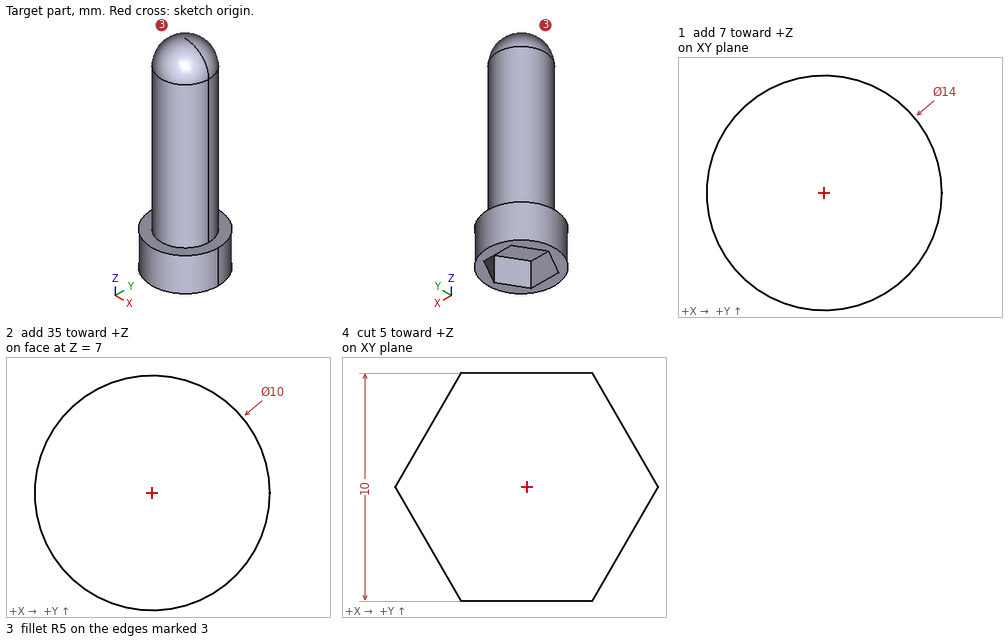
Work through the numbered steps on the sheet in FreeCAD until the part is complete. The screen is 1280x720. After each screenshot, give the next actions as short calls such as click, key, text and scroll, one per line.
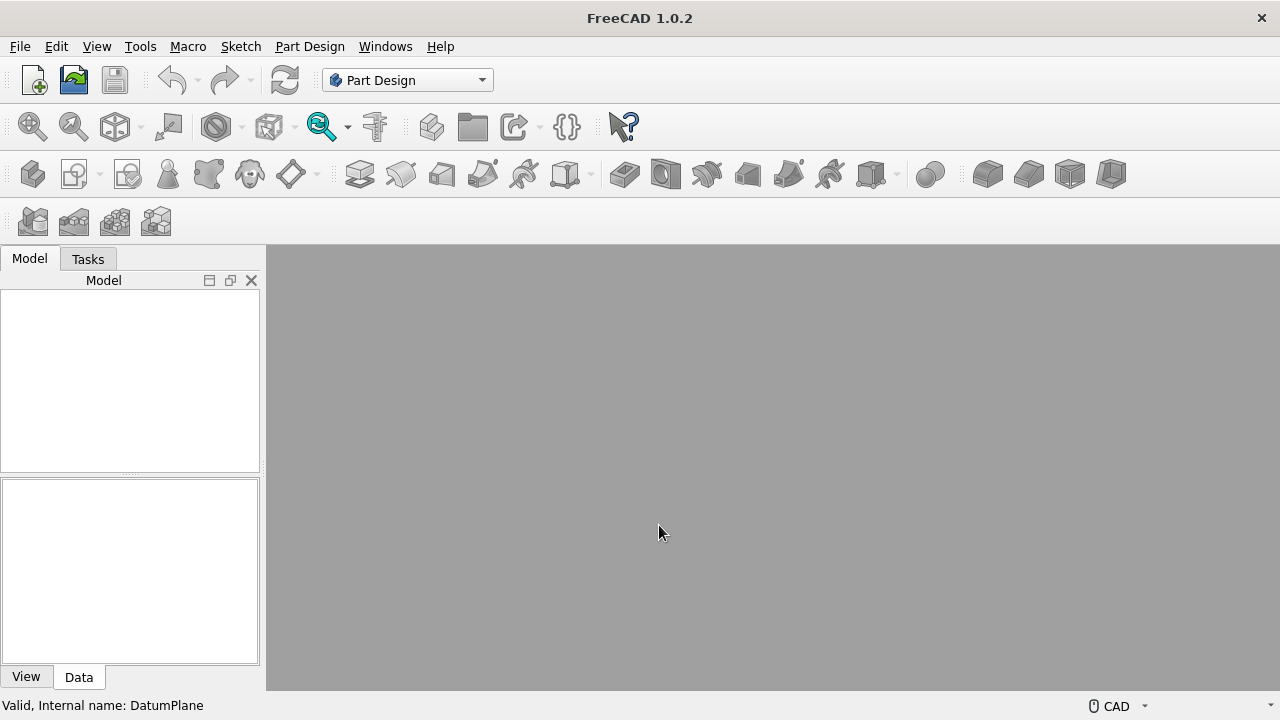
key(ctrl+n)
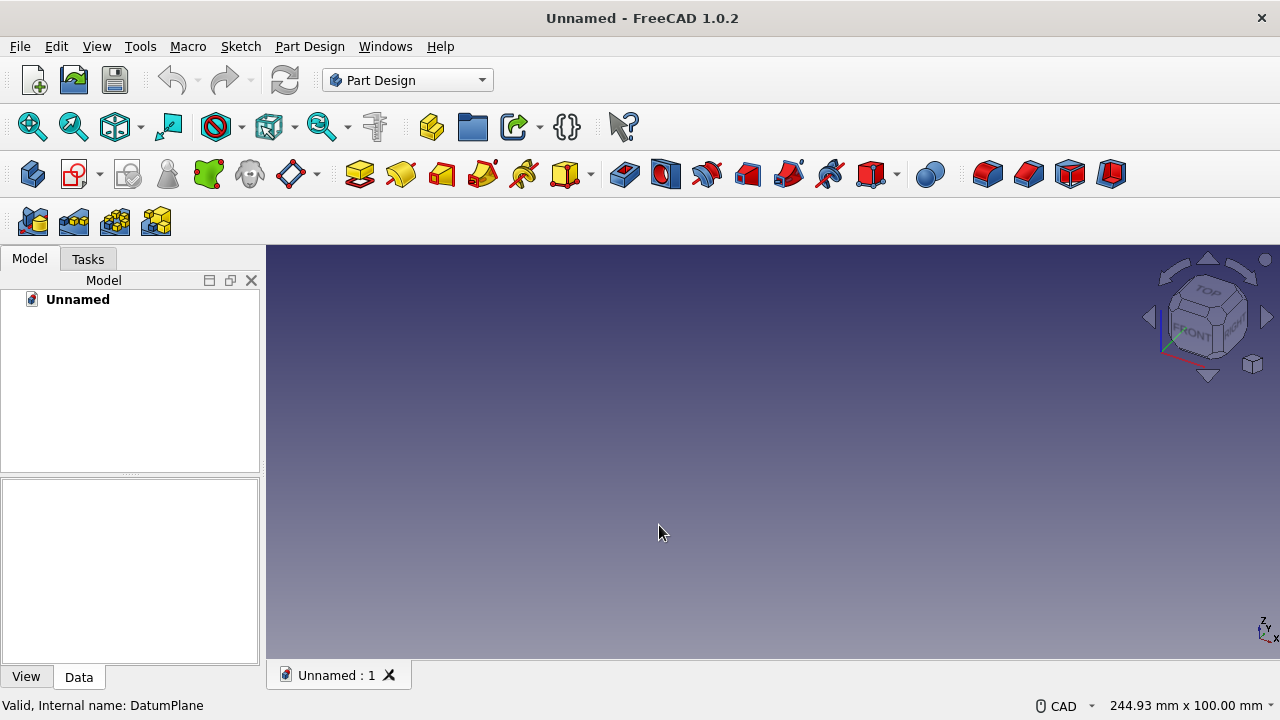
click(74, 174)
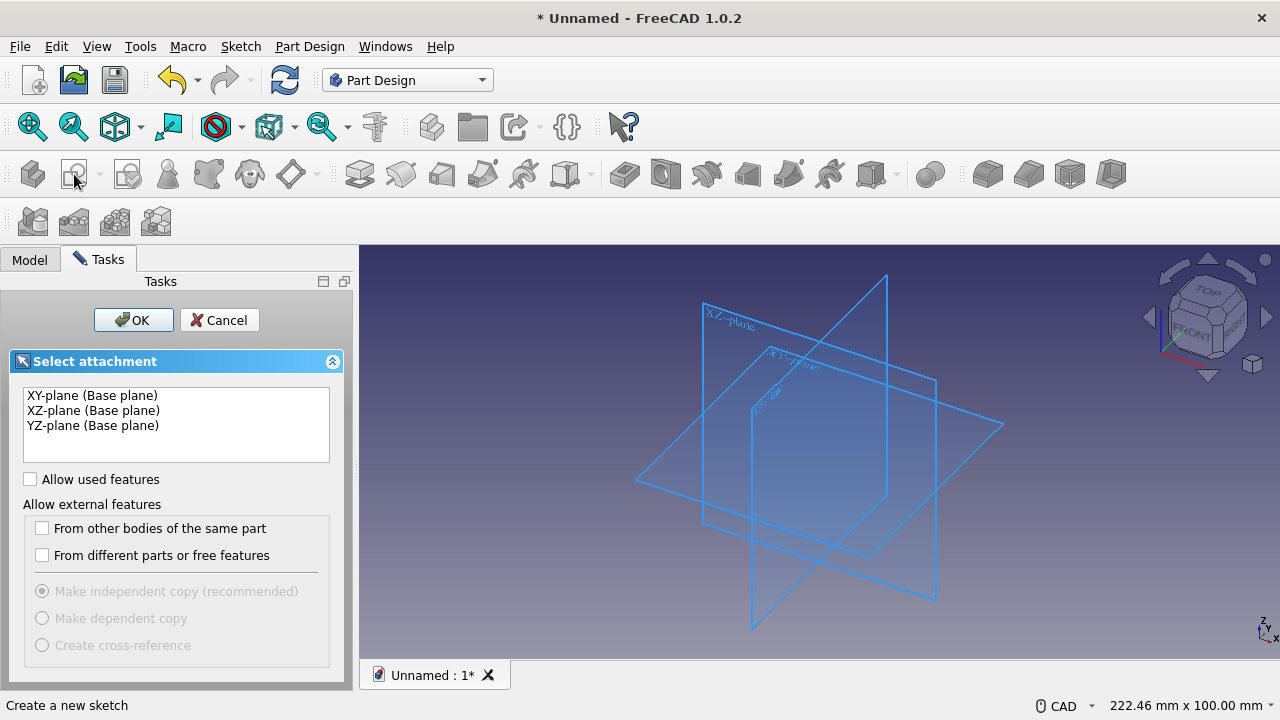
click(84, 396)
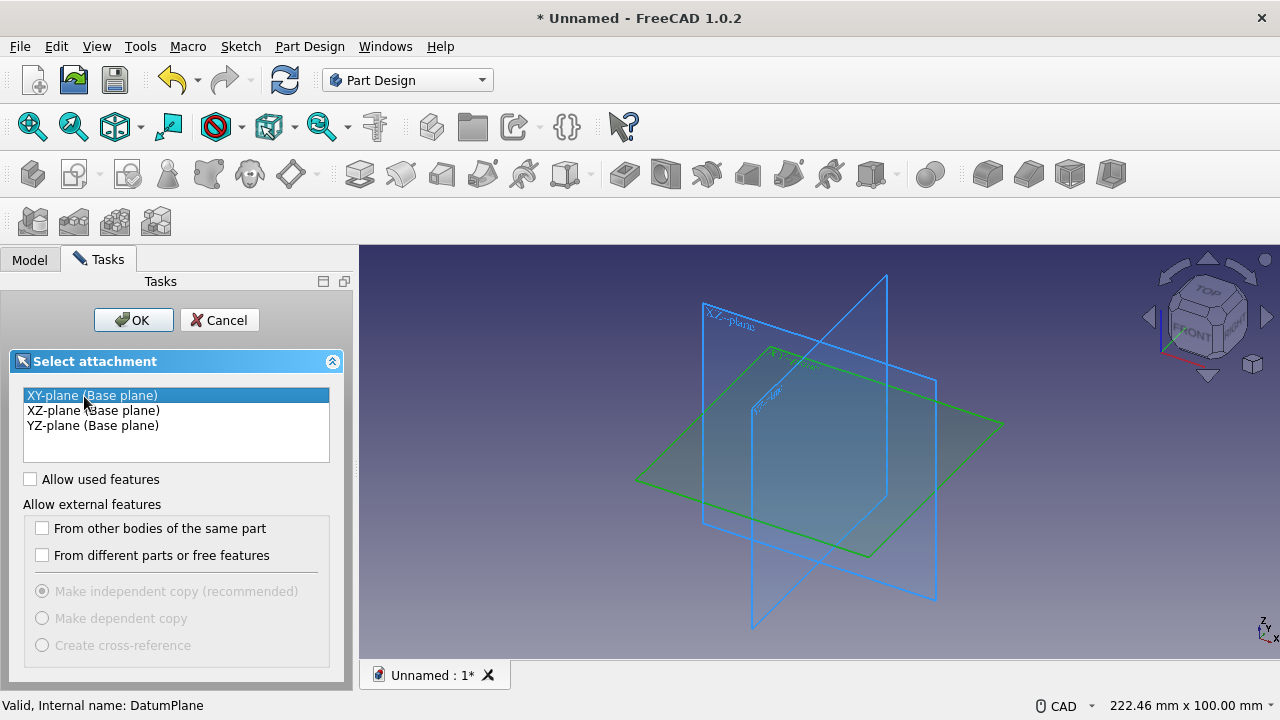
click(134, 320)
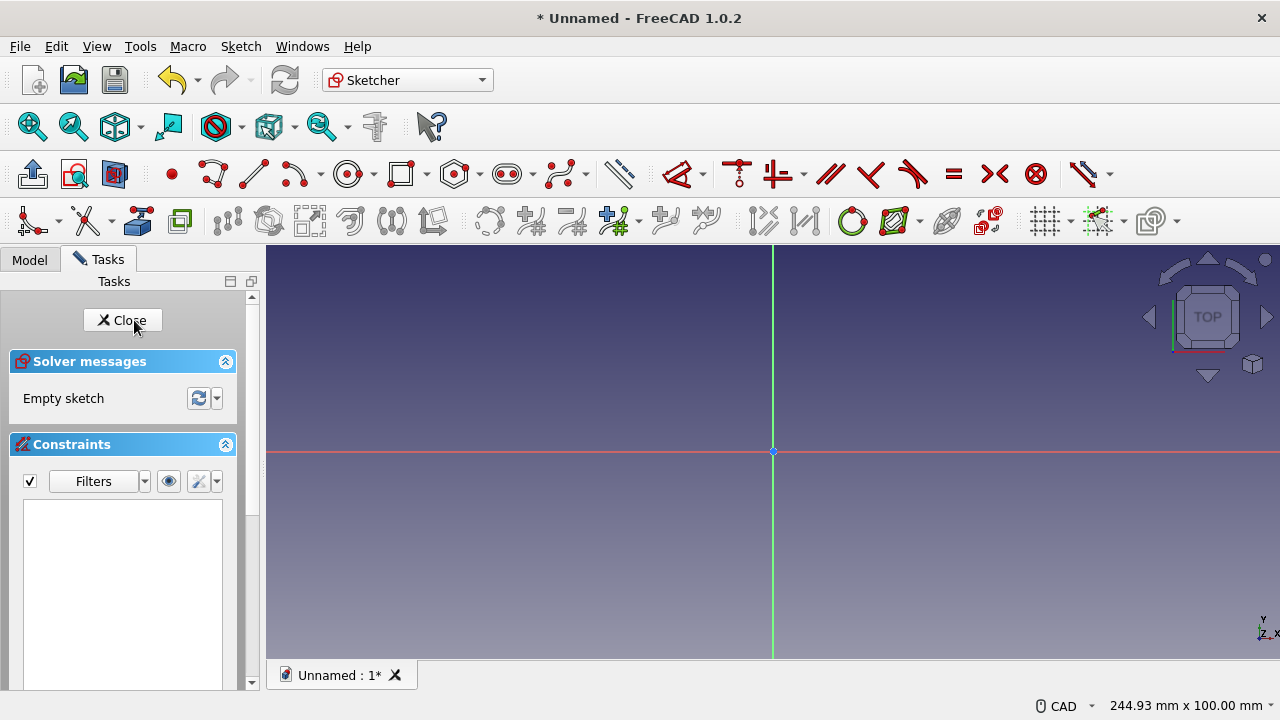
scroll(795, 452, up, 7)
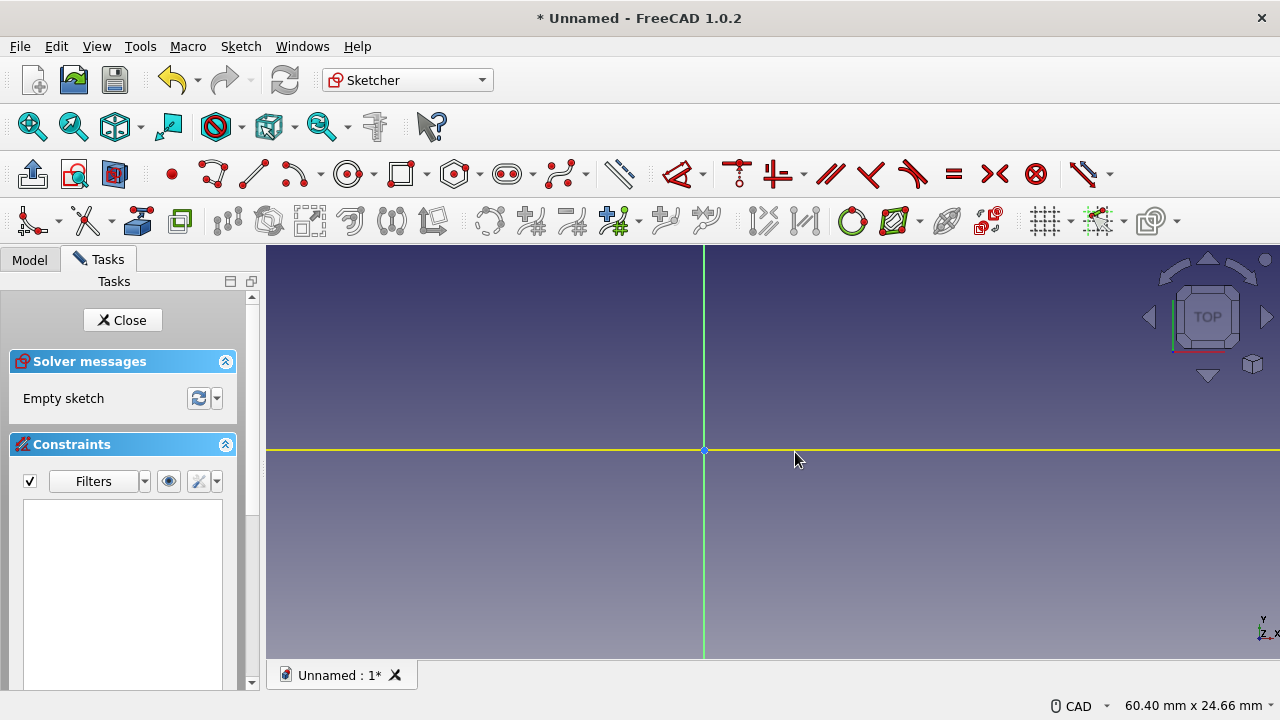
key(g)
key(c)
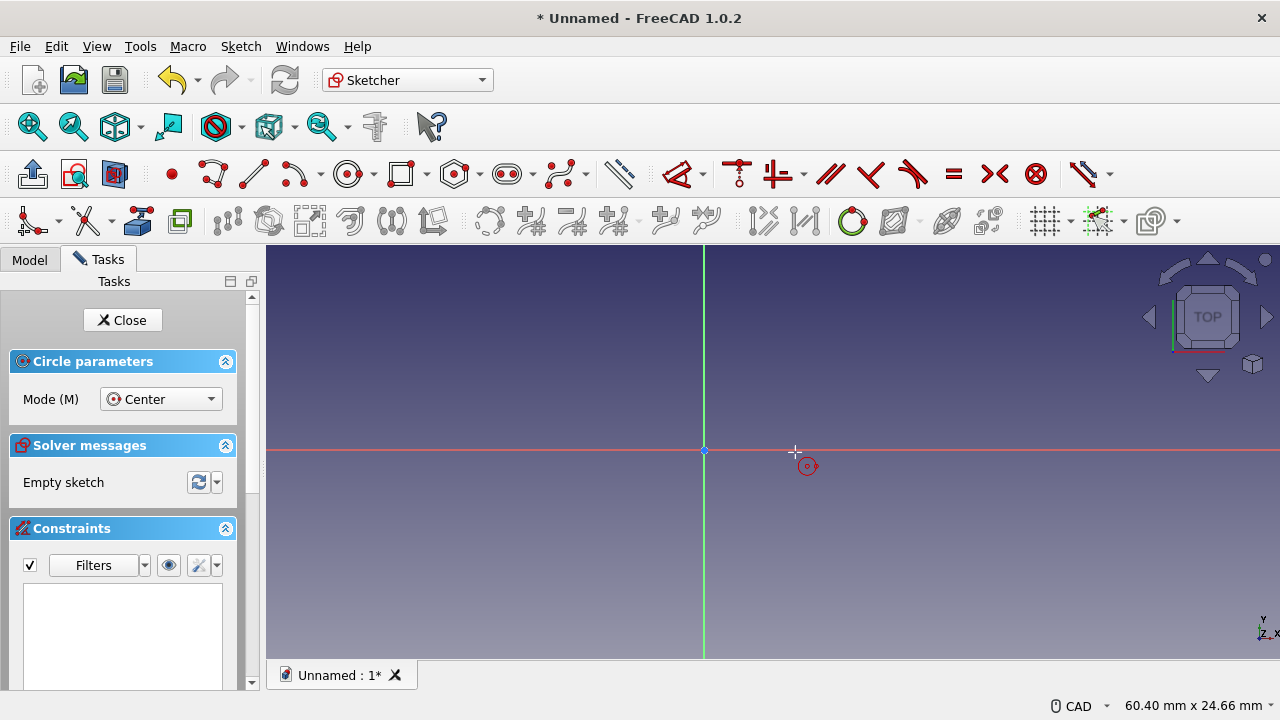
click(704, 450)
move(787, 367)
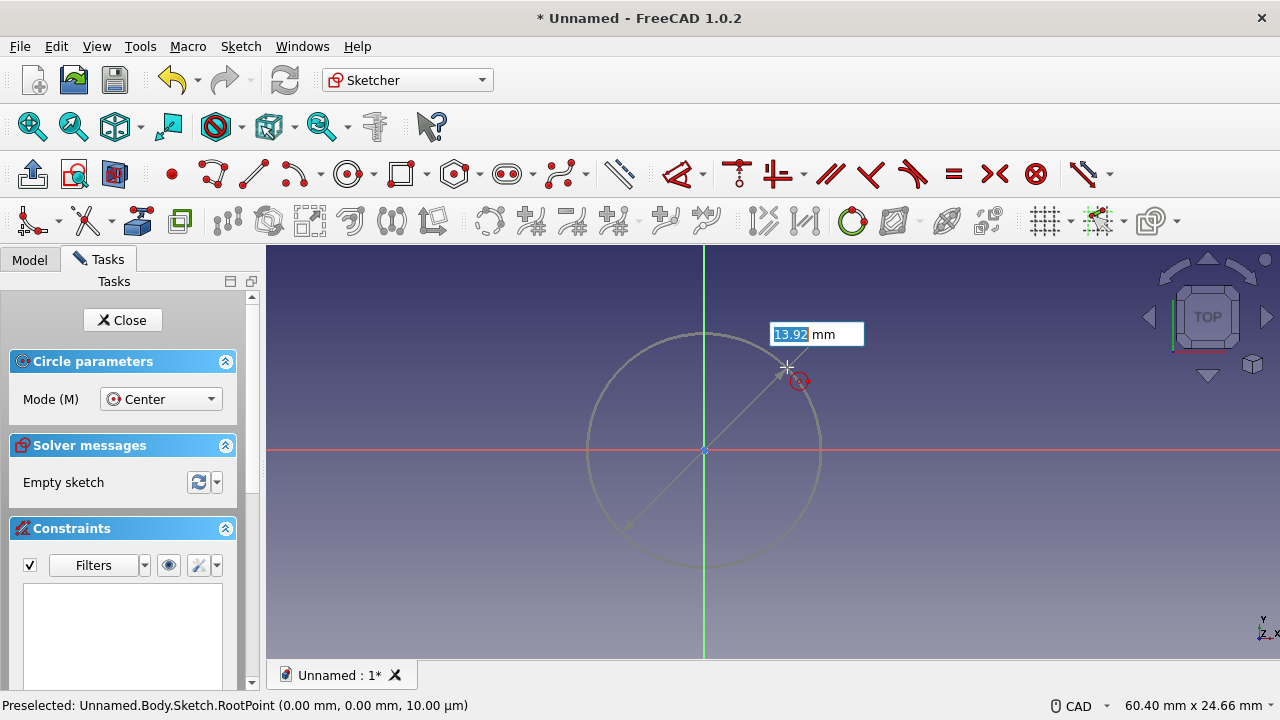
text(14)
key(Return)
key(Escape)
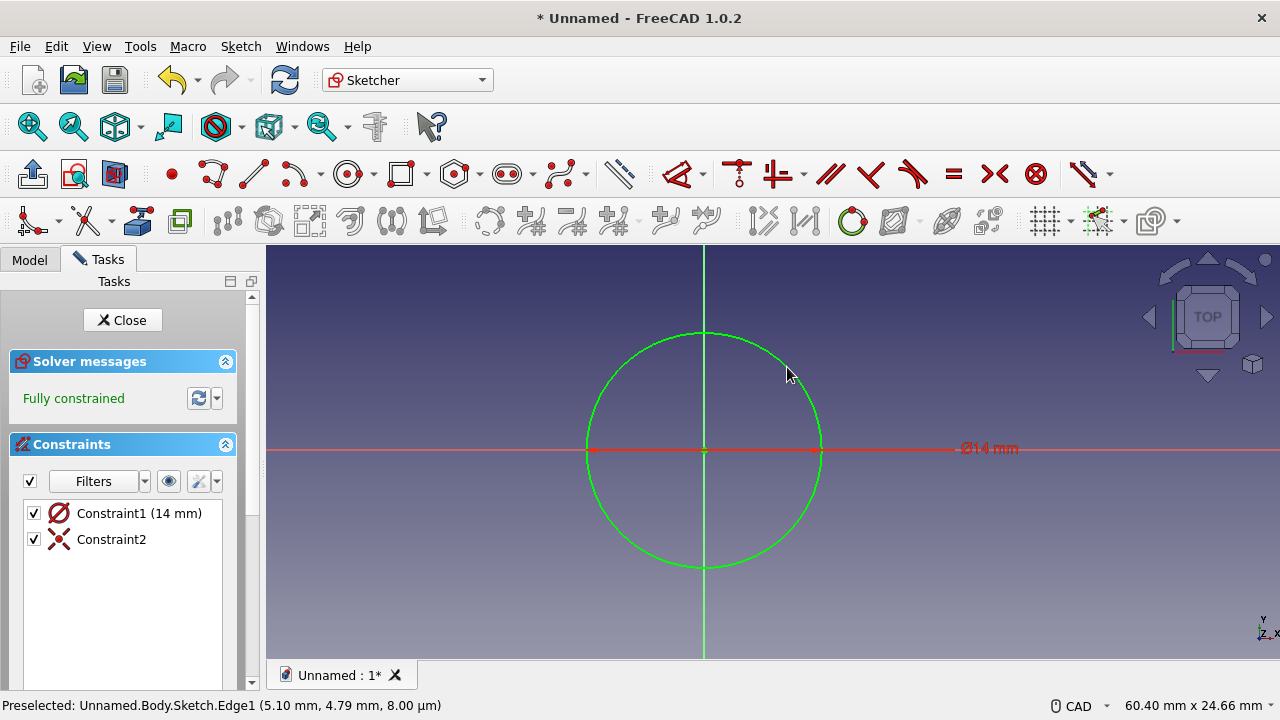
click(123, 320)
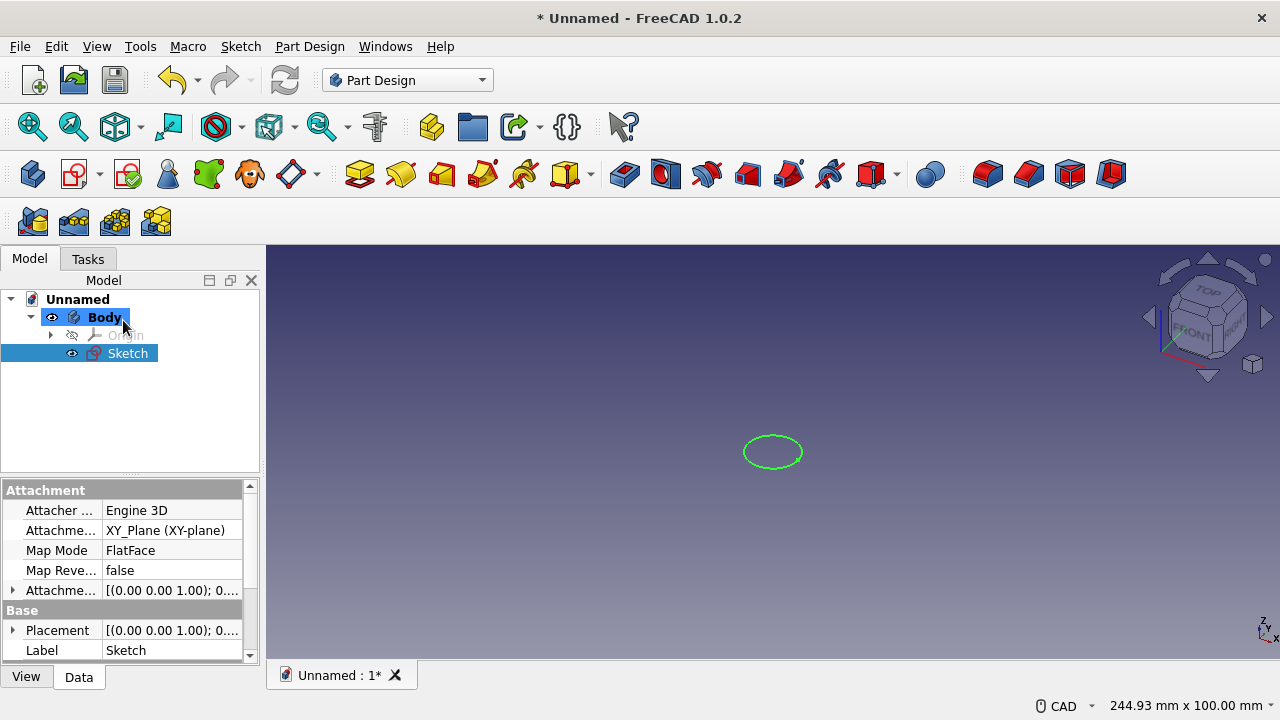
click(360, 174)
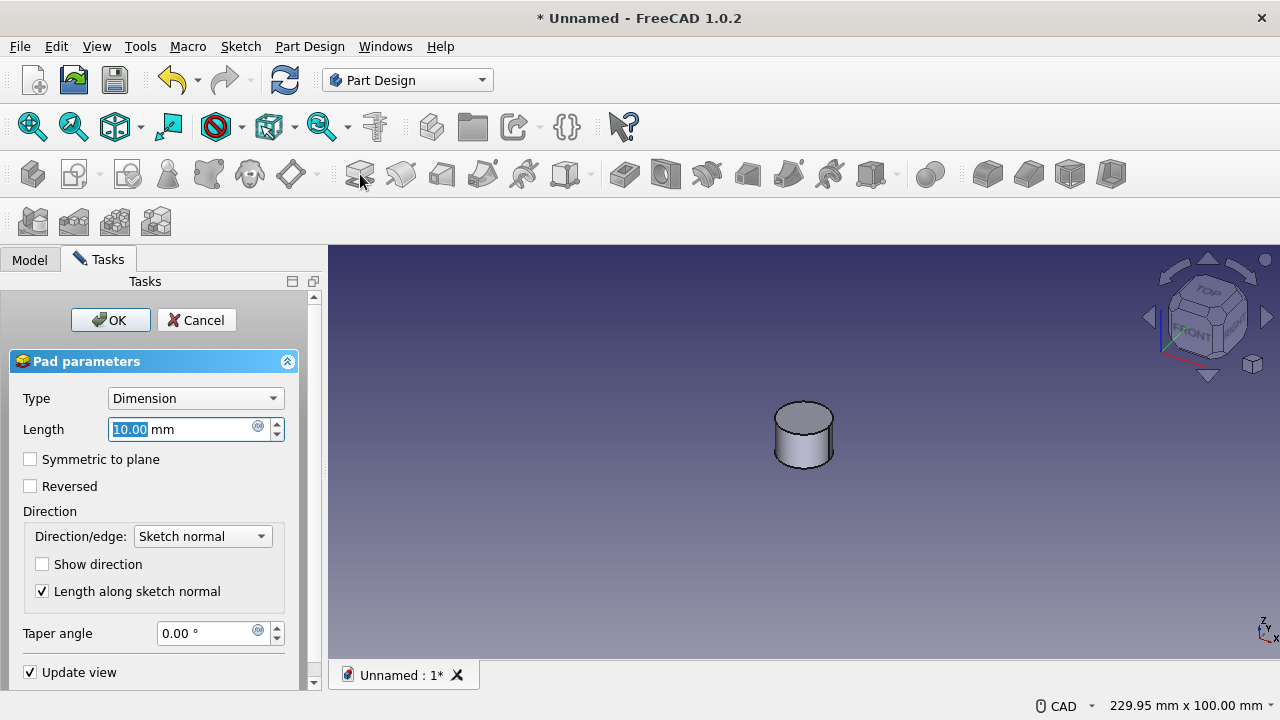
text(7)
key(Tab)